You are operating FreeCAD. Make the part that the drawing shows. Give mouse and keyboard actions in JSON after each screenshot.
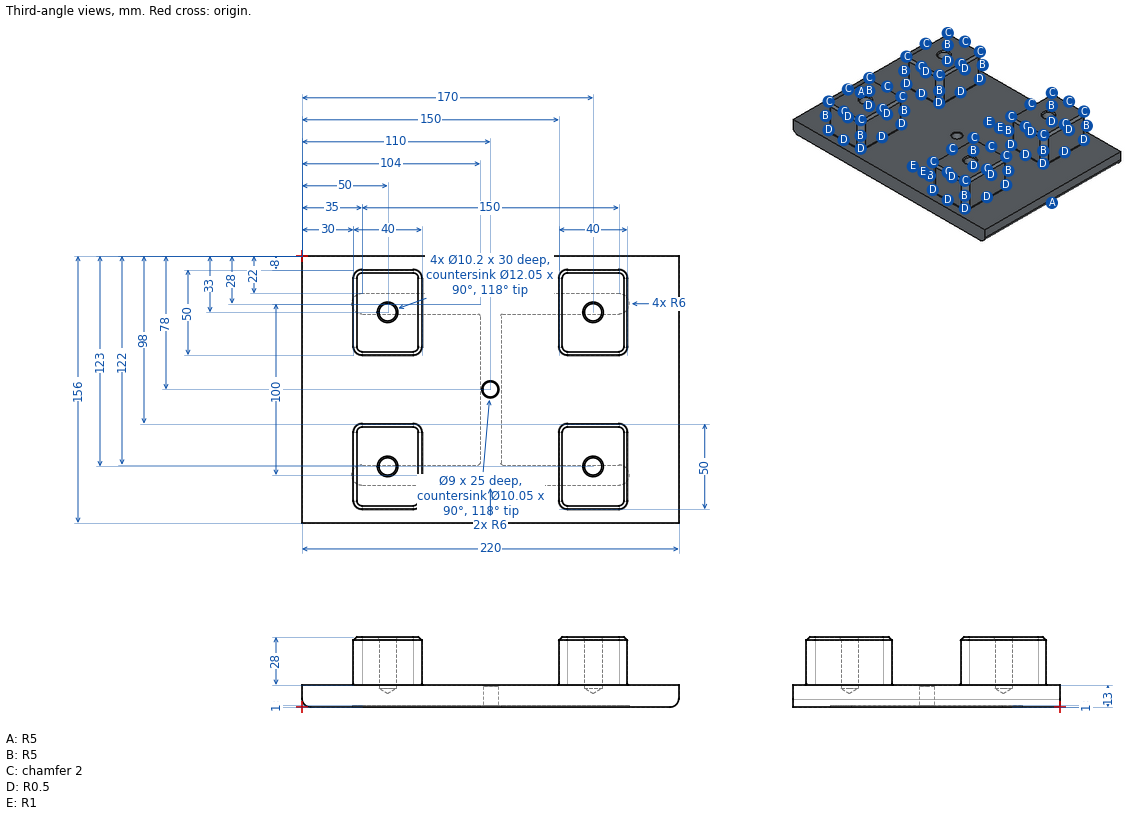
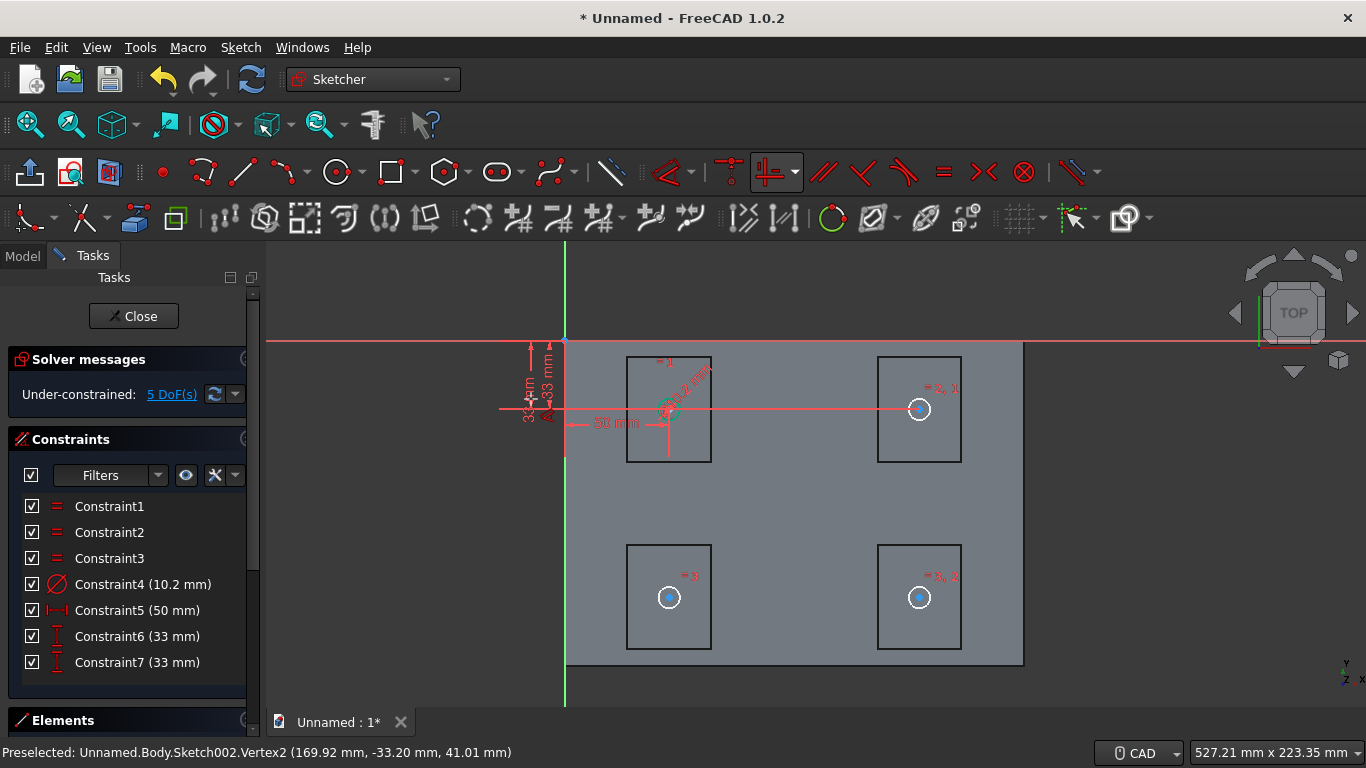
{"action": "left_click", "coordinate": [669, 598]}
{"action": "left_click", "coordinate": [617, 307]}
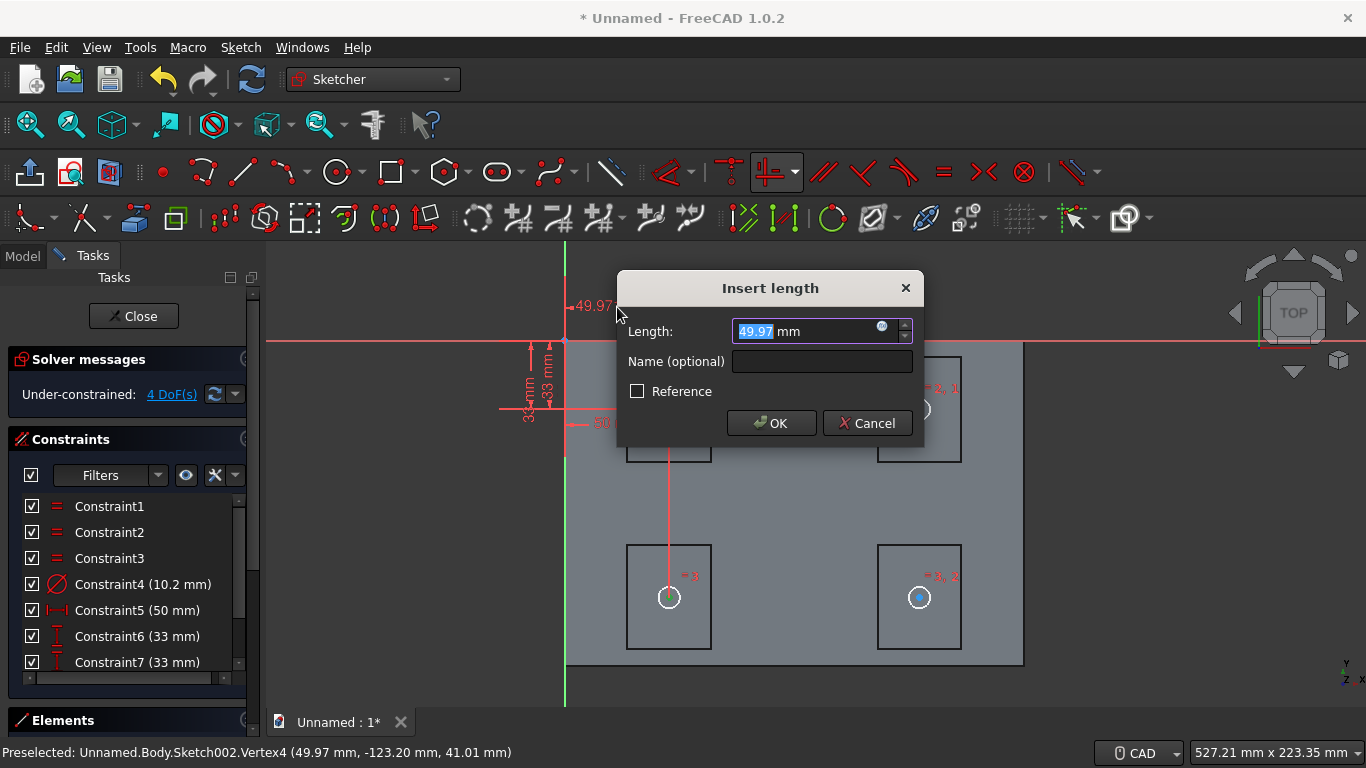
{"action": "type", "text": "50"}
{"action": "key", "text": "Return"}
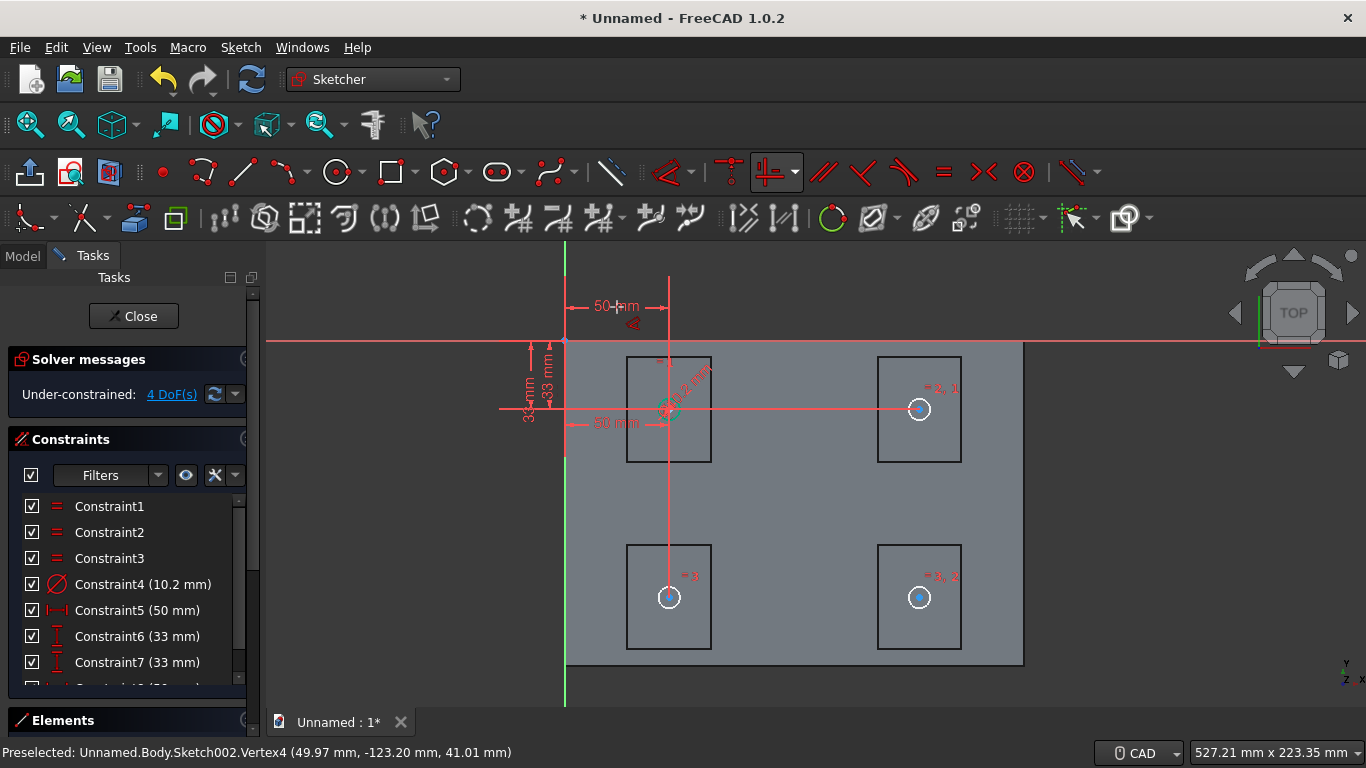
{"action": "left_click", "coordinate": [919, 409]}
{"action": "left_click", "coordinate": [742, 307]}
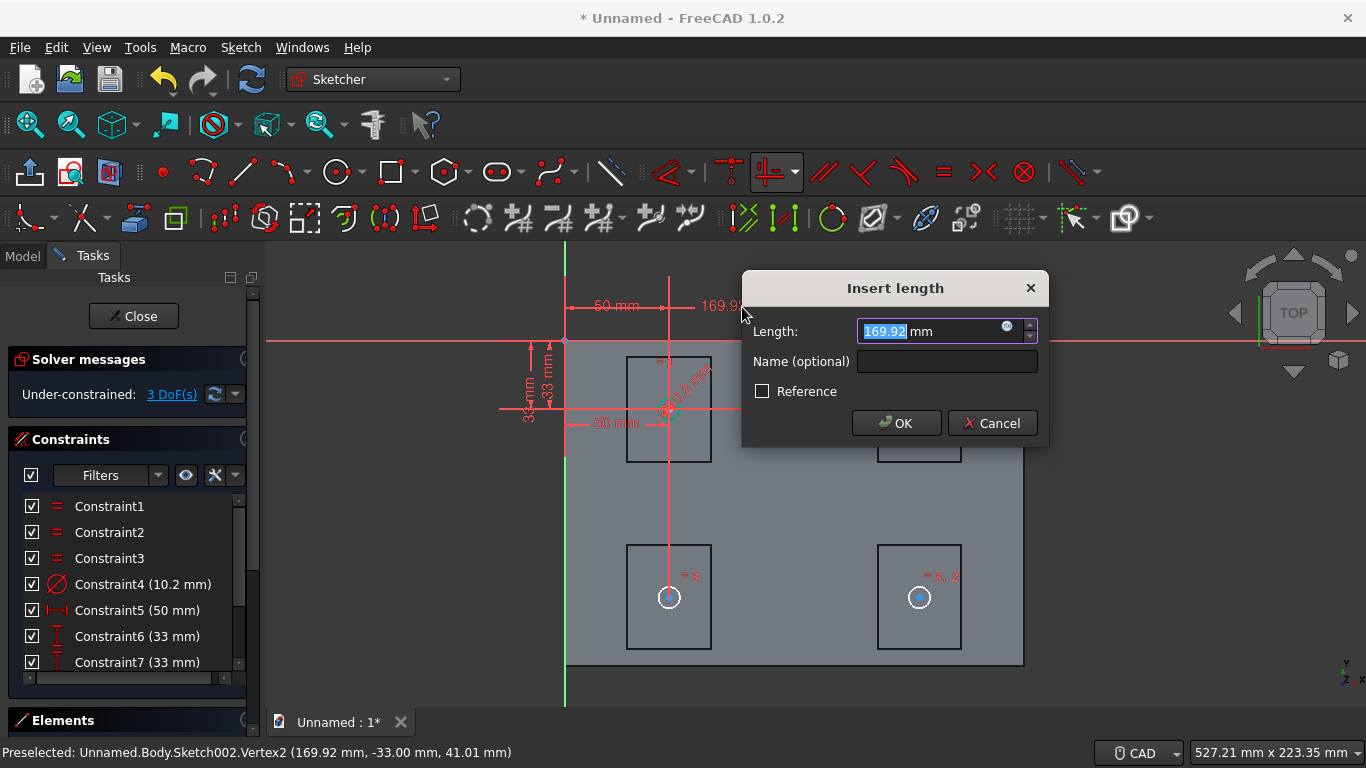
{"action": "type", "text": "170"}
{"action": "key", "text": "Return"}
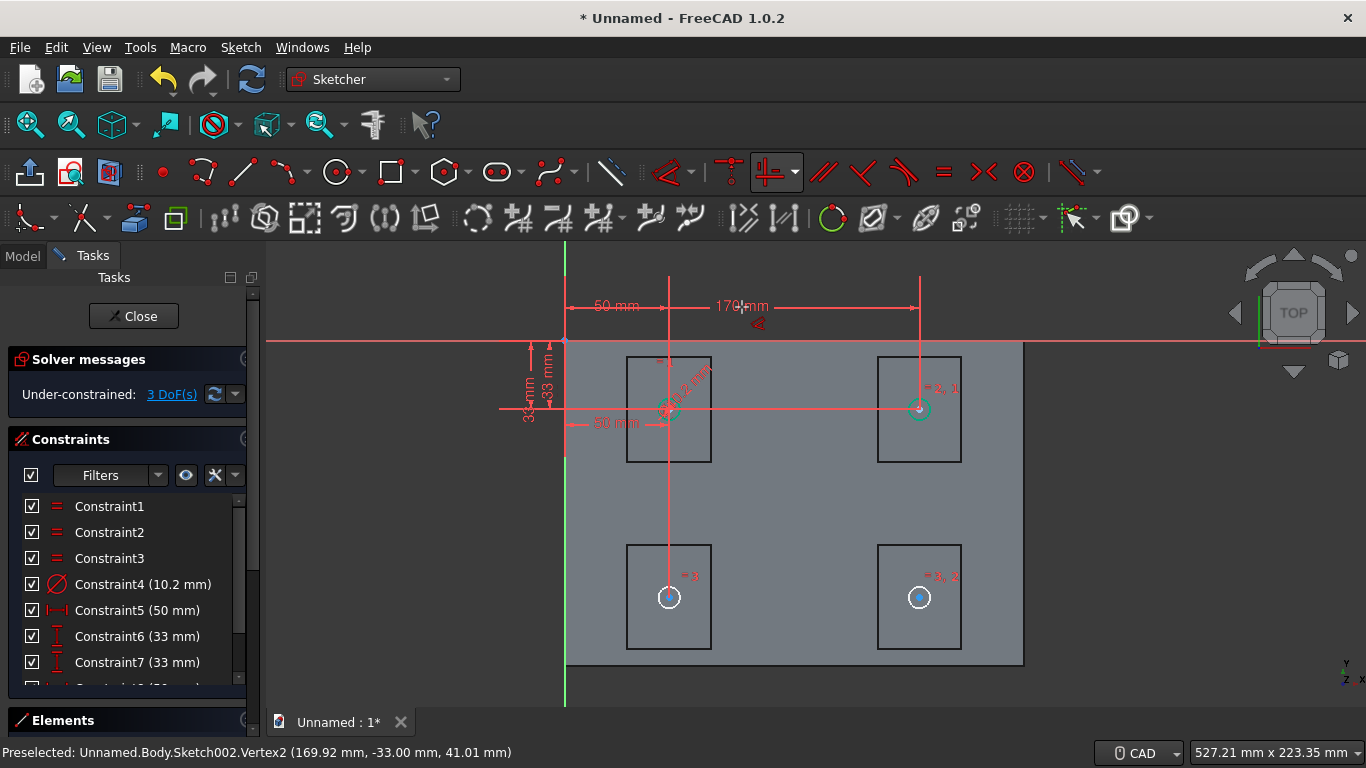
{"action": "left_click", "coordinate": [919, 598]}
{"action": "left_click", "coordinate": [824, 307]}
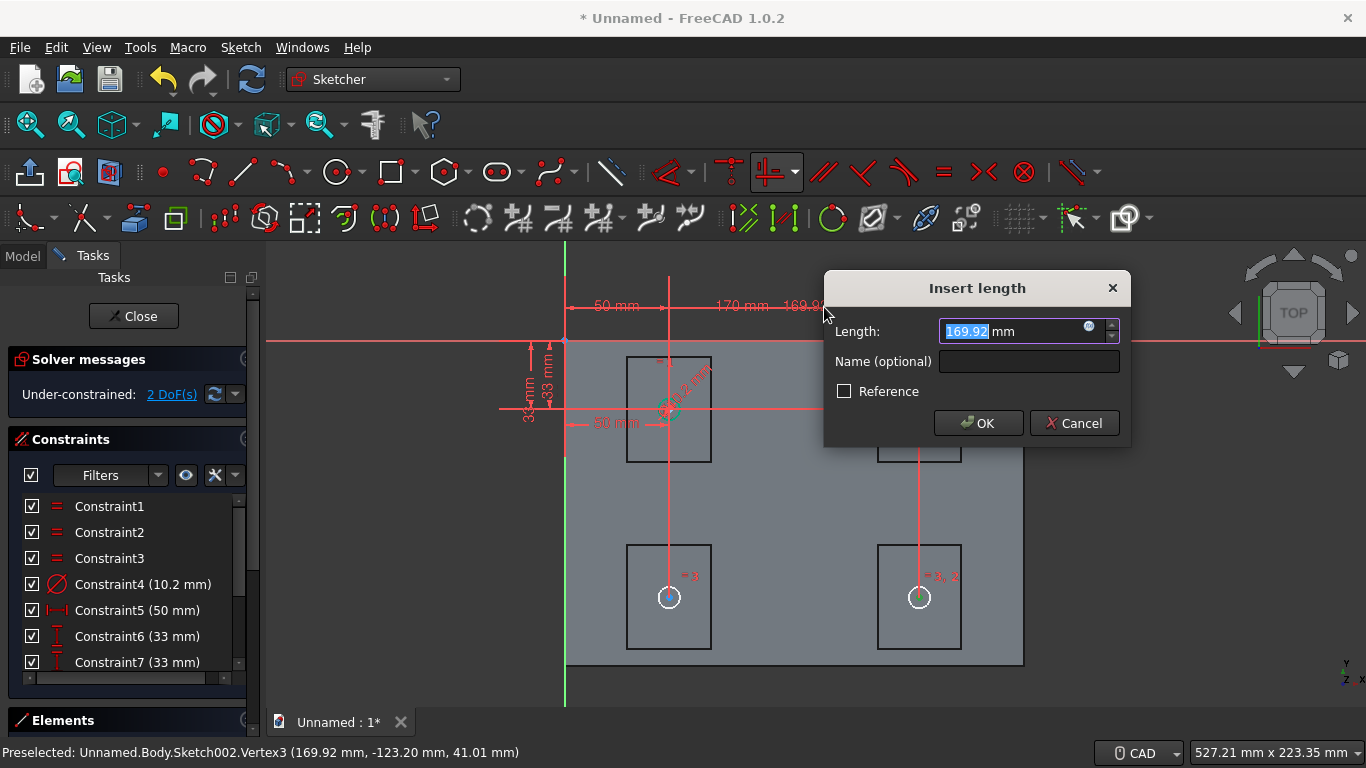
{"action": "type", "text": "170"}
{"action": "key", "text": "Return"}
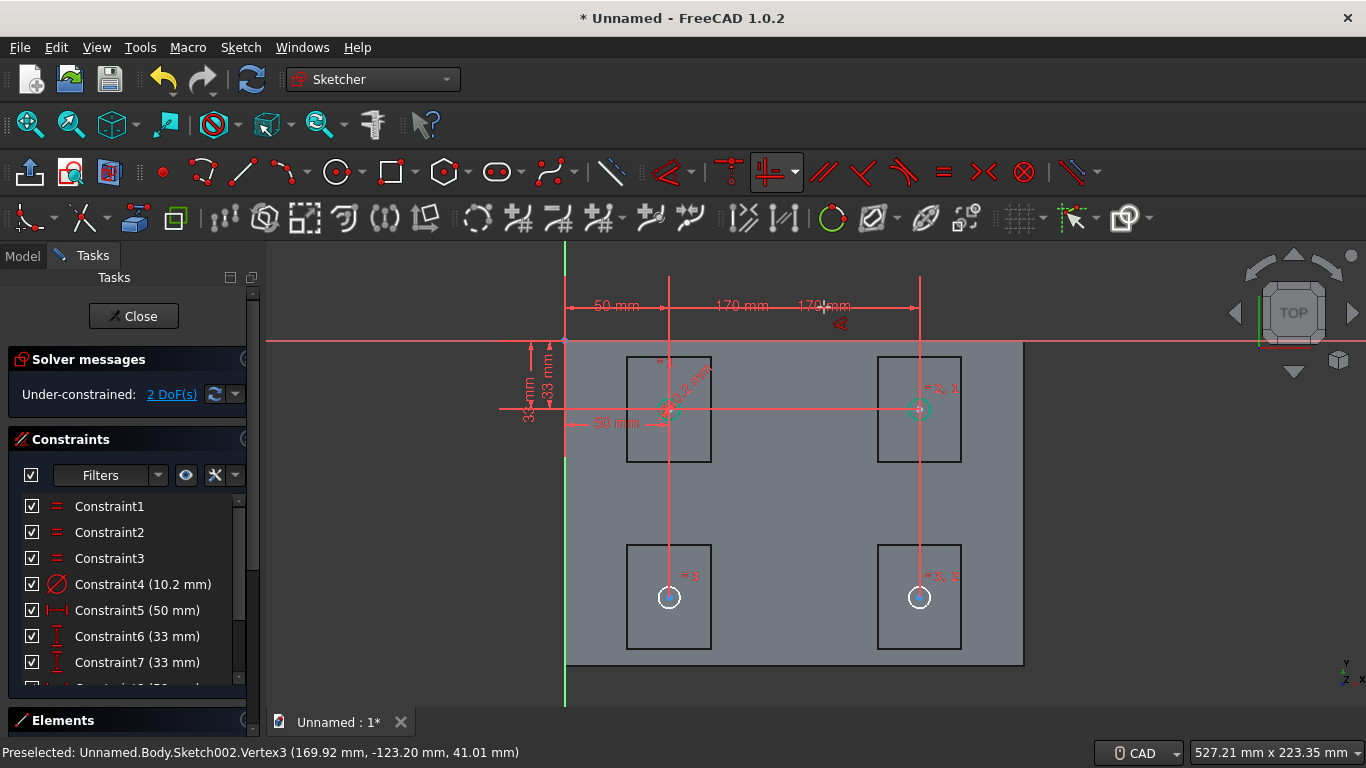
{"action": "left_click", "coordinate": [920, 598]}
{"action": "left_click", "coordinate": [531, 469]}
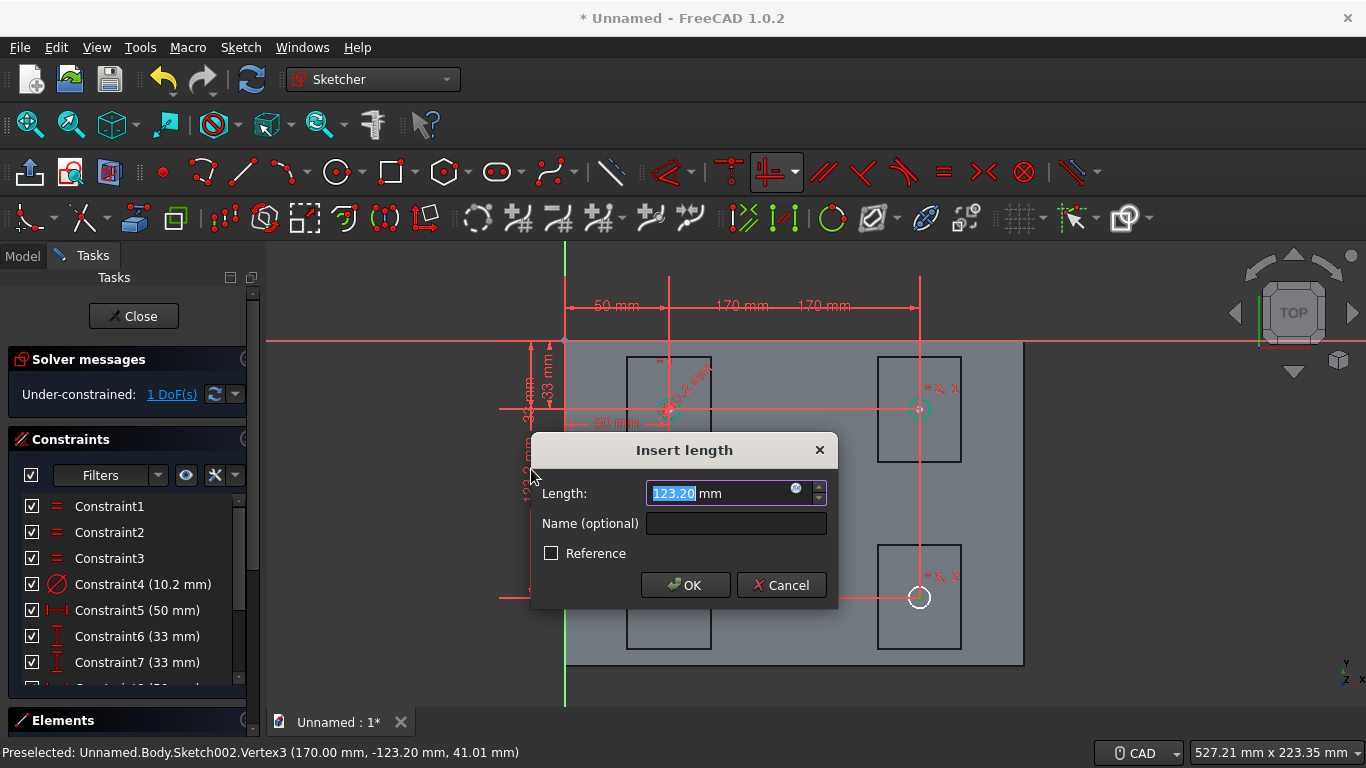
{"action": "type", "text": "123"}
{"action": "key", "text": "Return"}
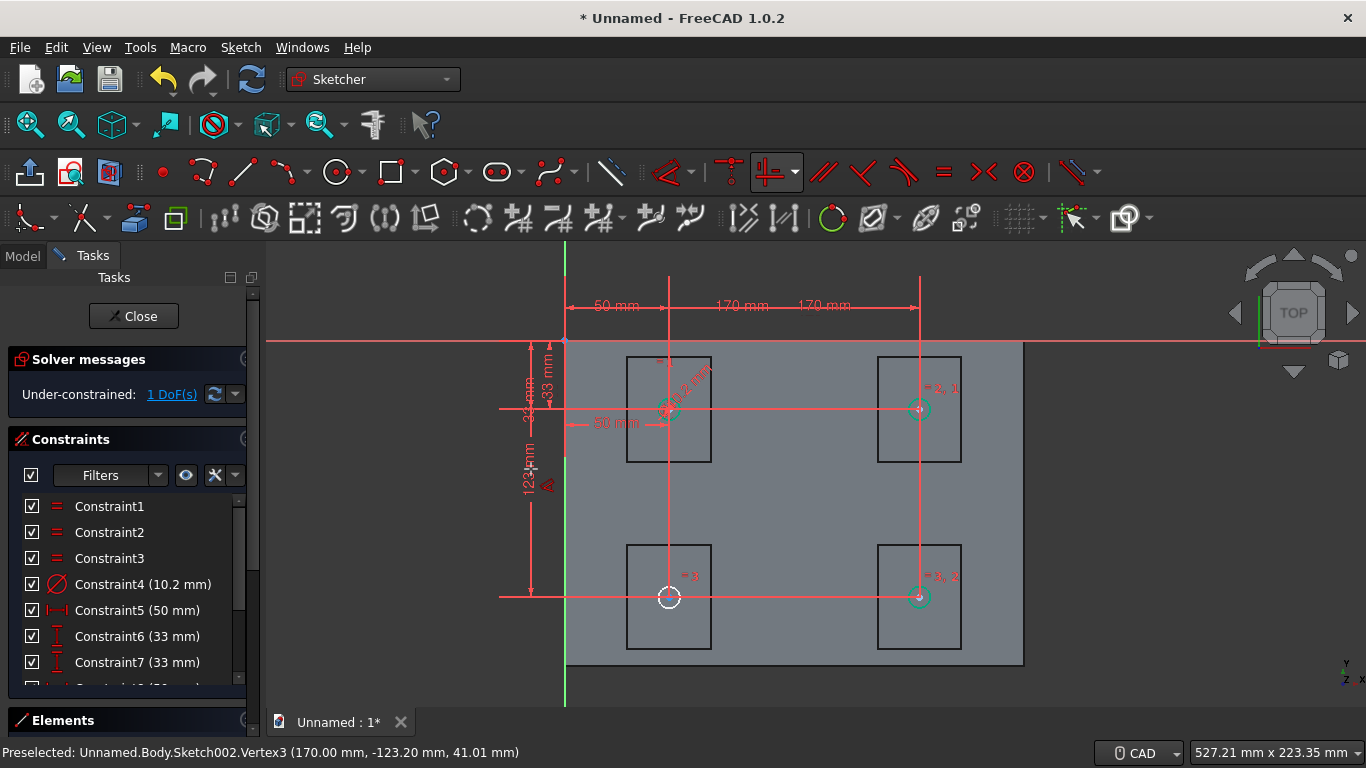
{"action": "left_click", "coordinate": [669, 598]}
{"action": "left_click", "coordinate": [531, 528]}